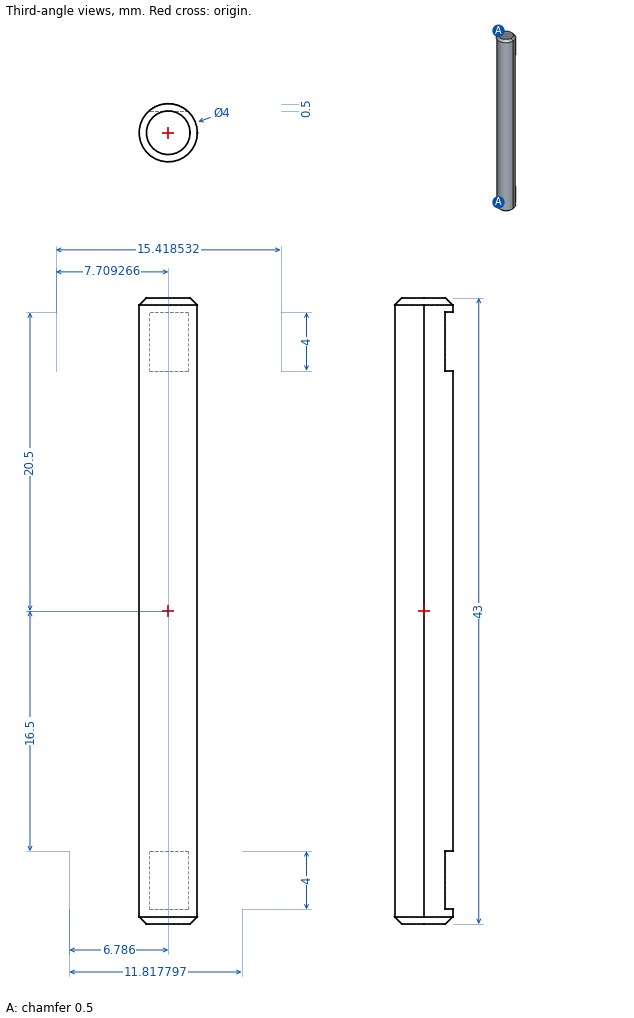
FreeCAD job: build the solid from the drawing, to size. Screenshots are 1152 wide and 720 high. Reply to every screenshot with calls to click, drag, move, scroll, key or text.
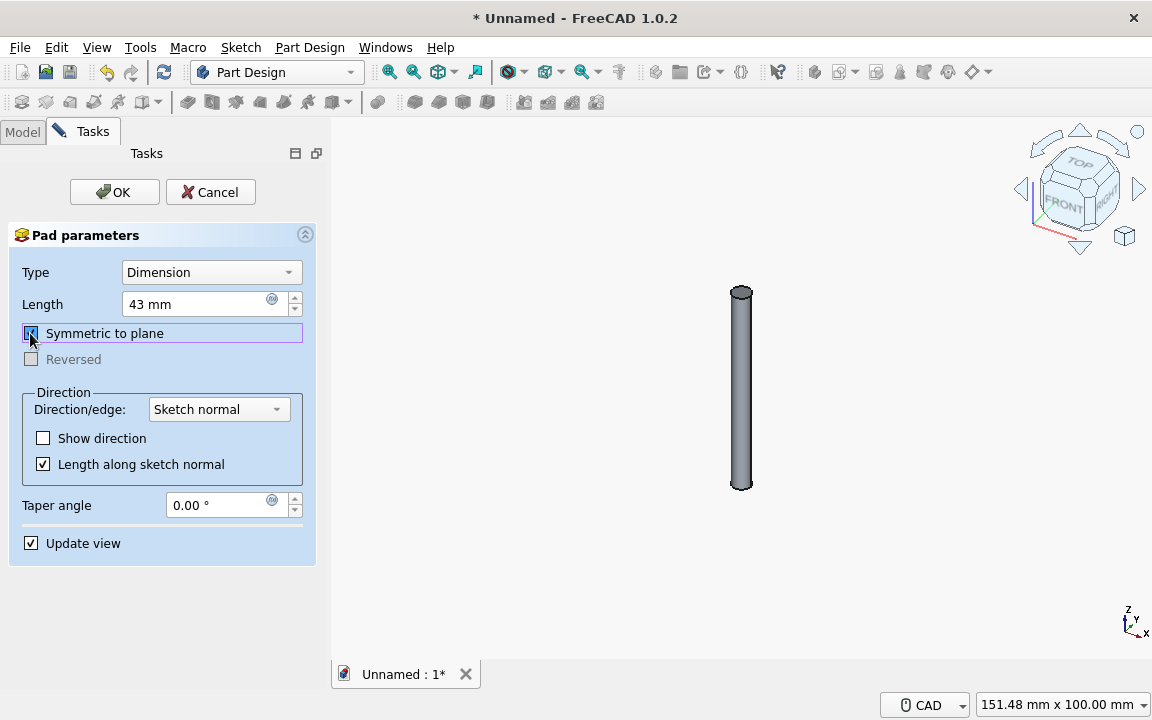
click(115, 192)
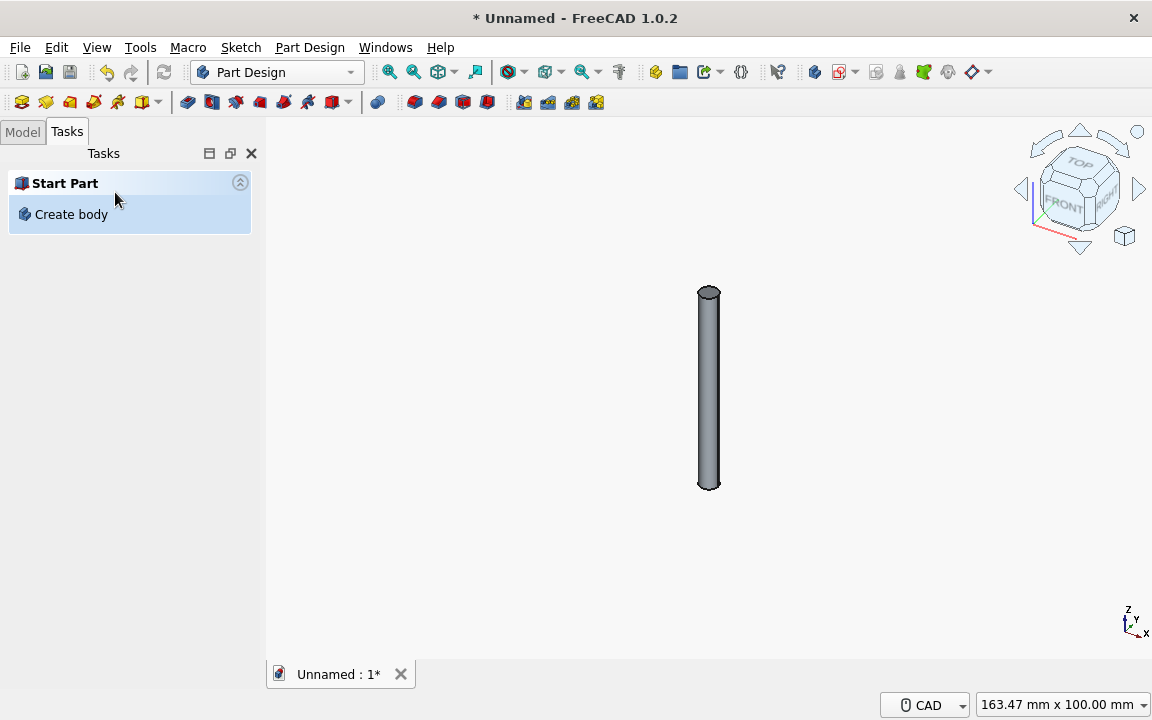
key(v)
key(f)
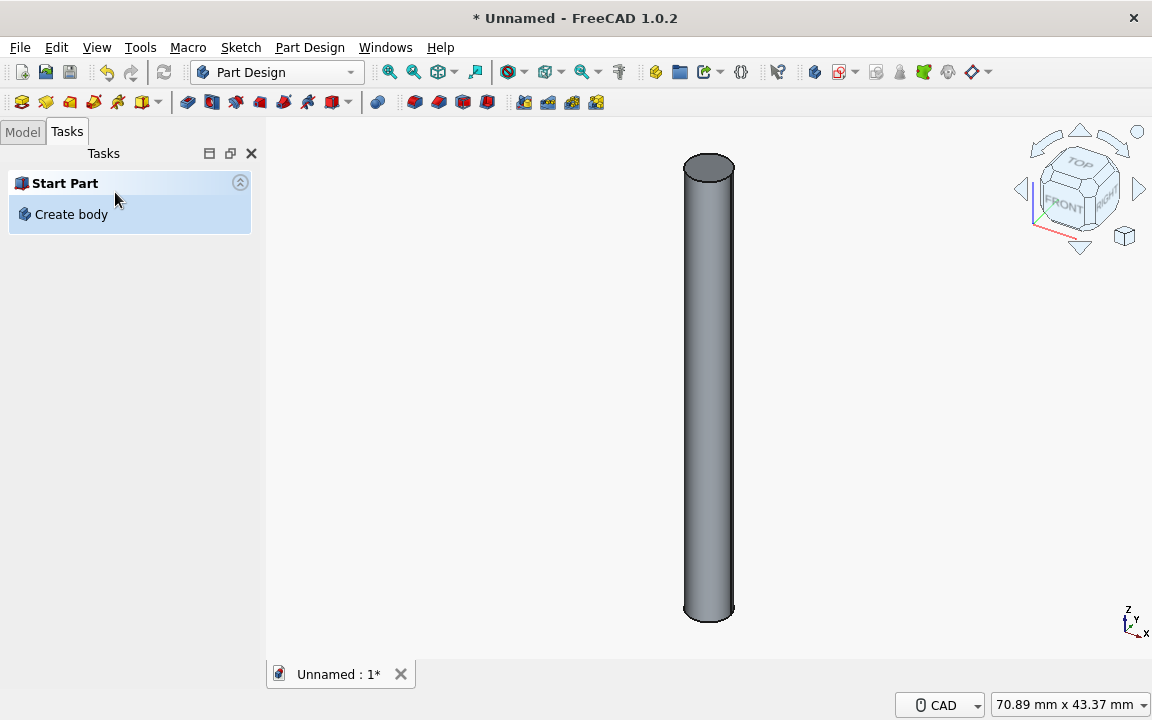
click(23, 131)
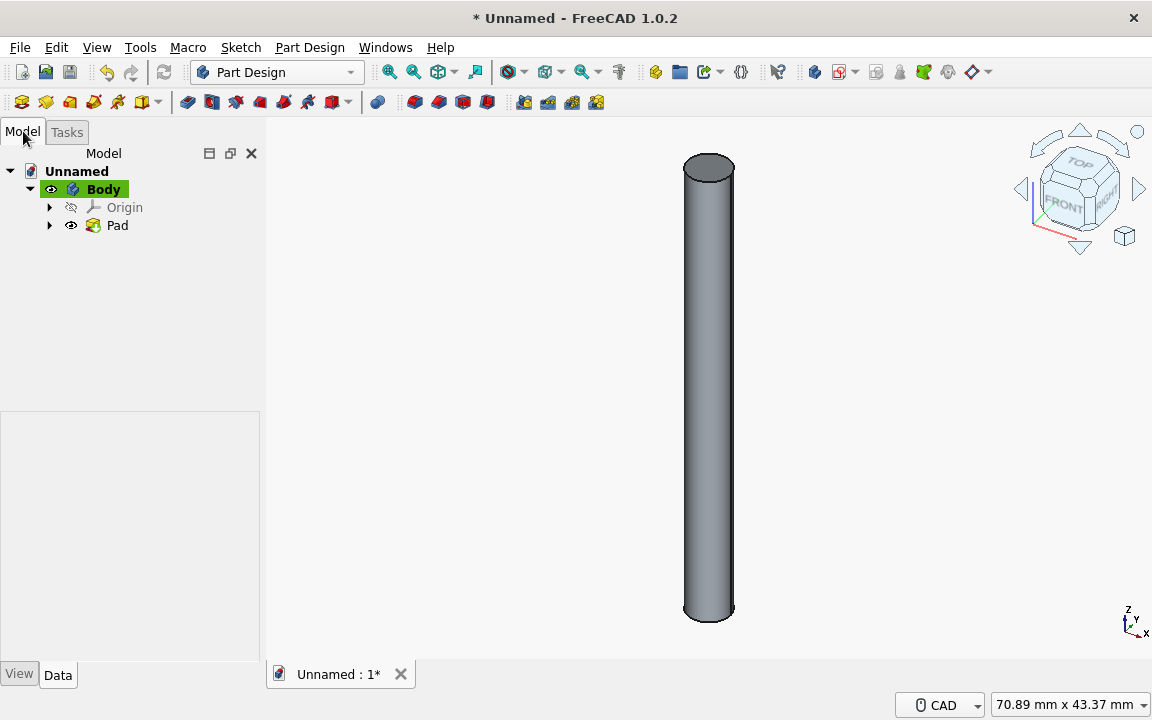
click(50, 207)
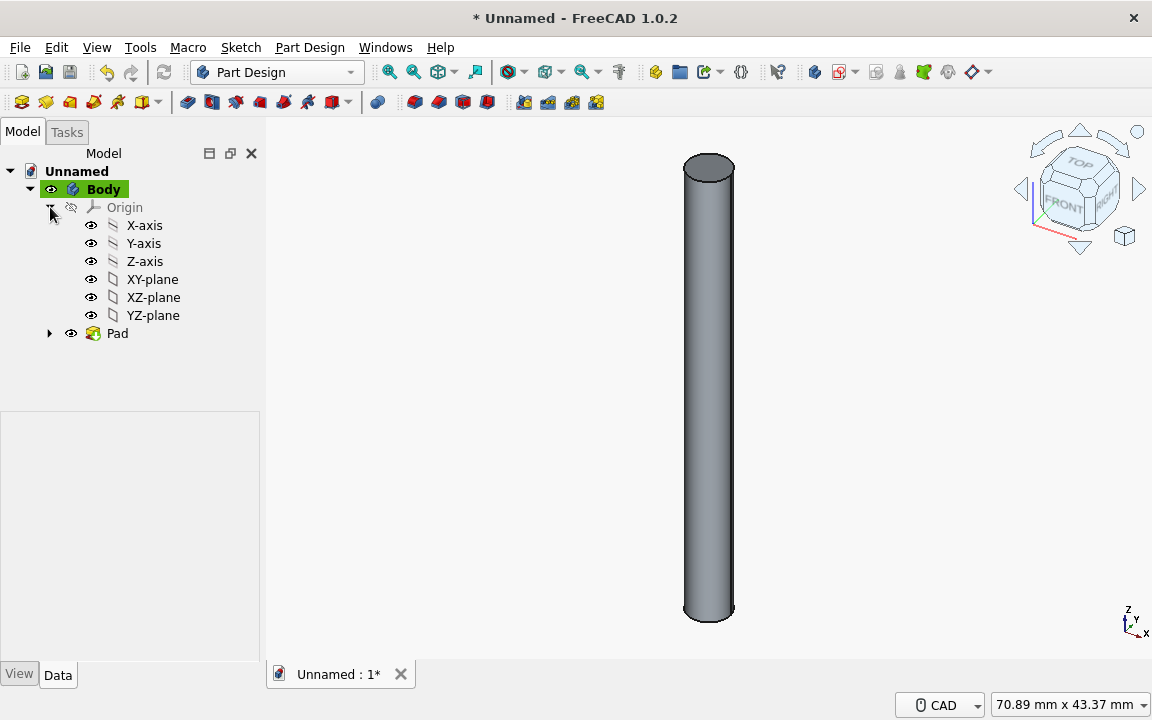
click(136, 297)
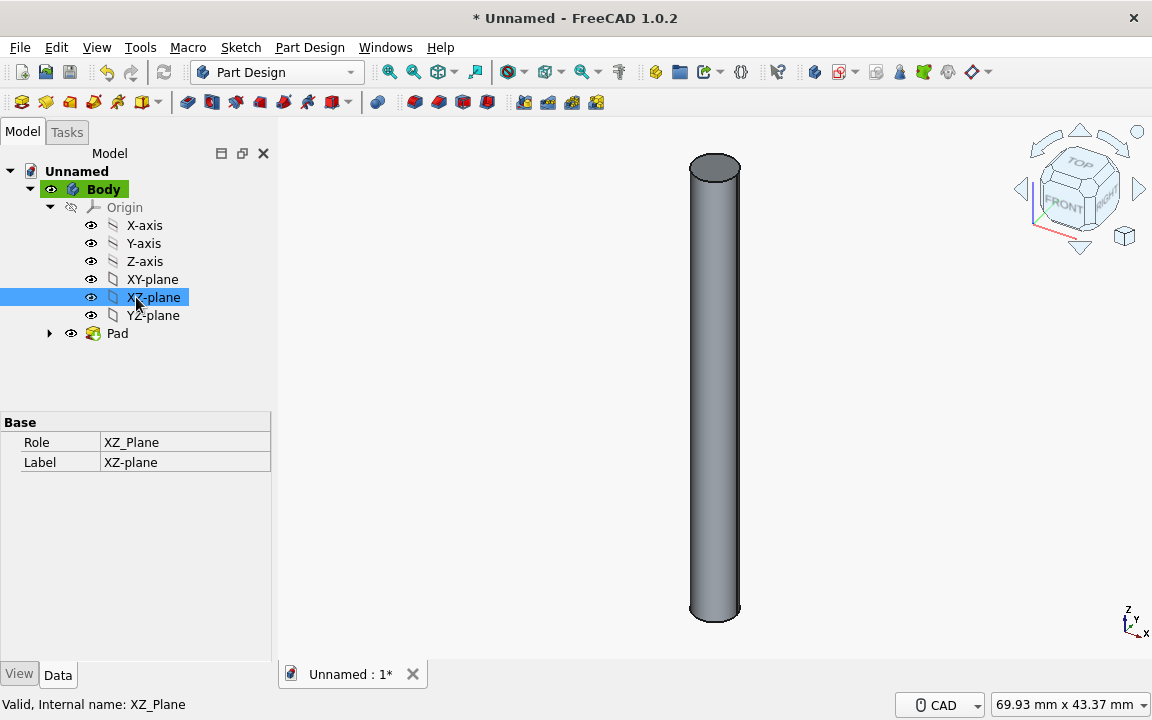
click(972, 72)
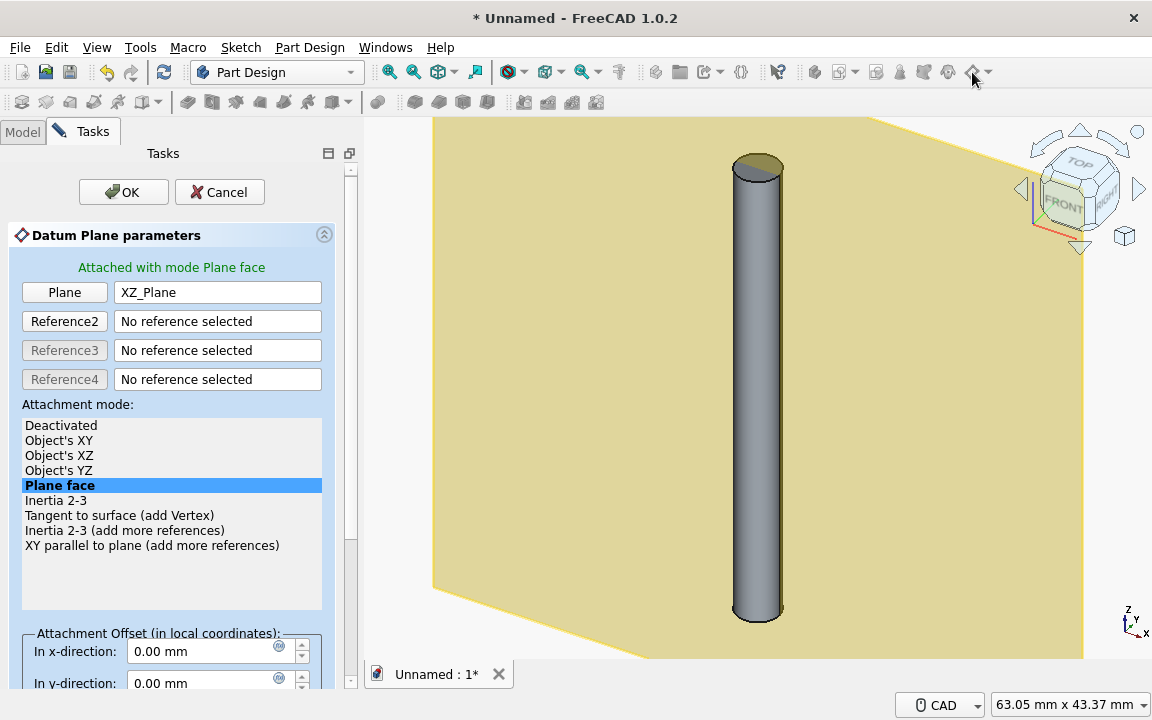
scroll(351, 426, down, 2)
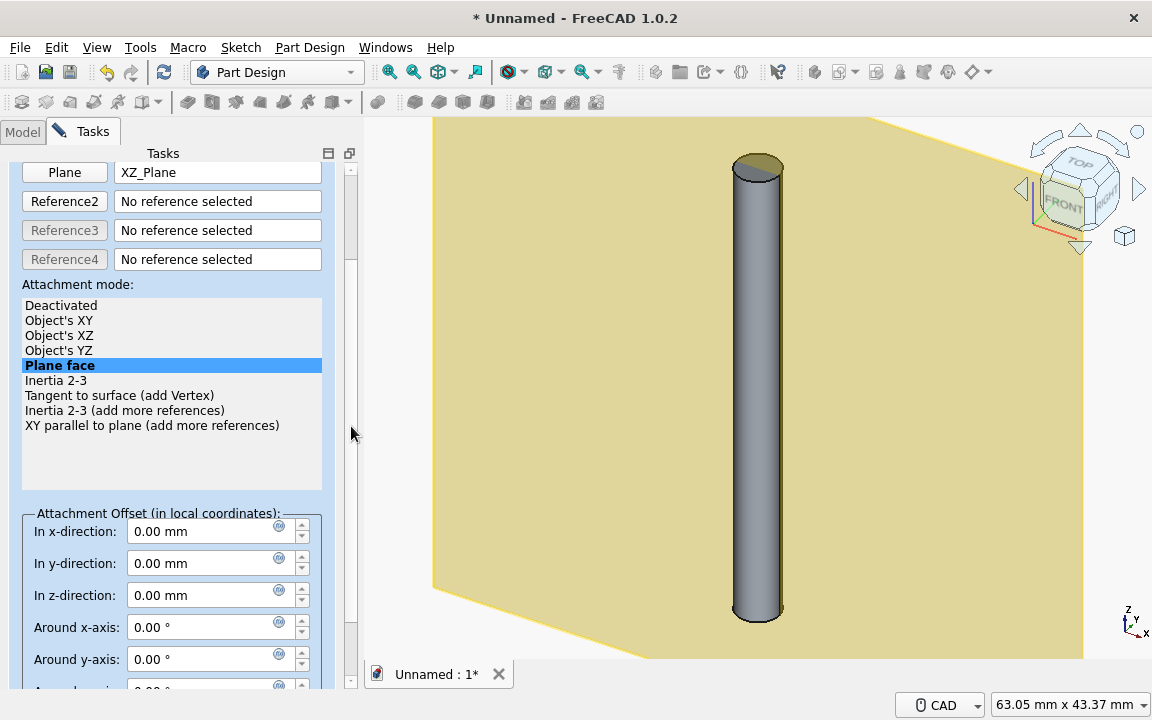
triple_click(210, 595)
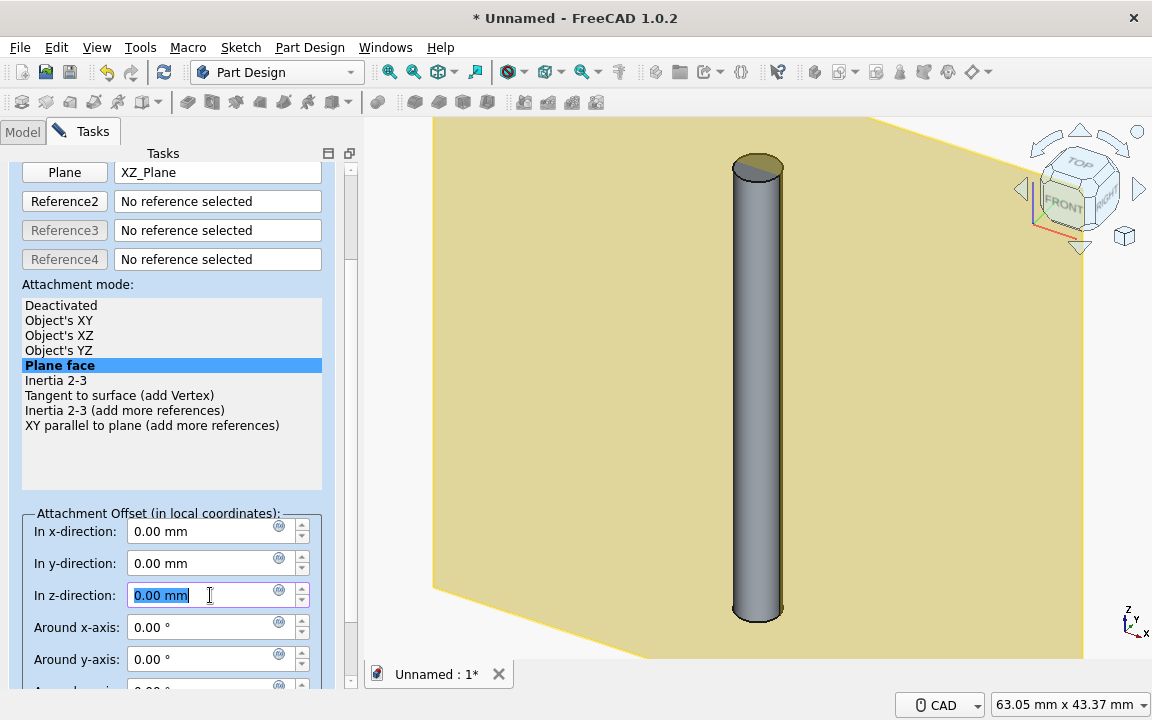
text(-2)
key(Tab)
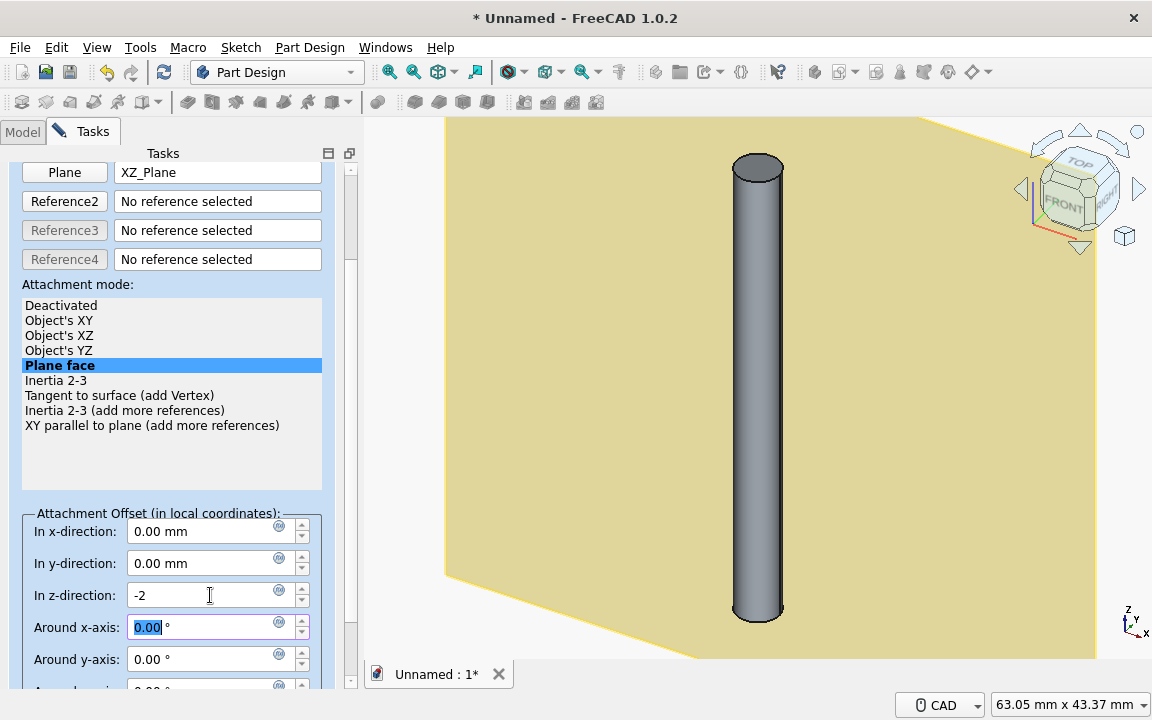
scroll(351, 426, up, 3)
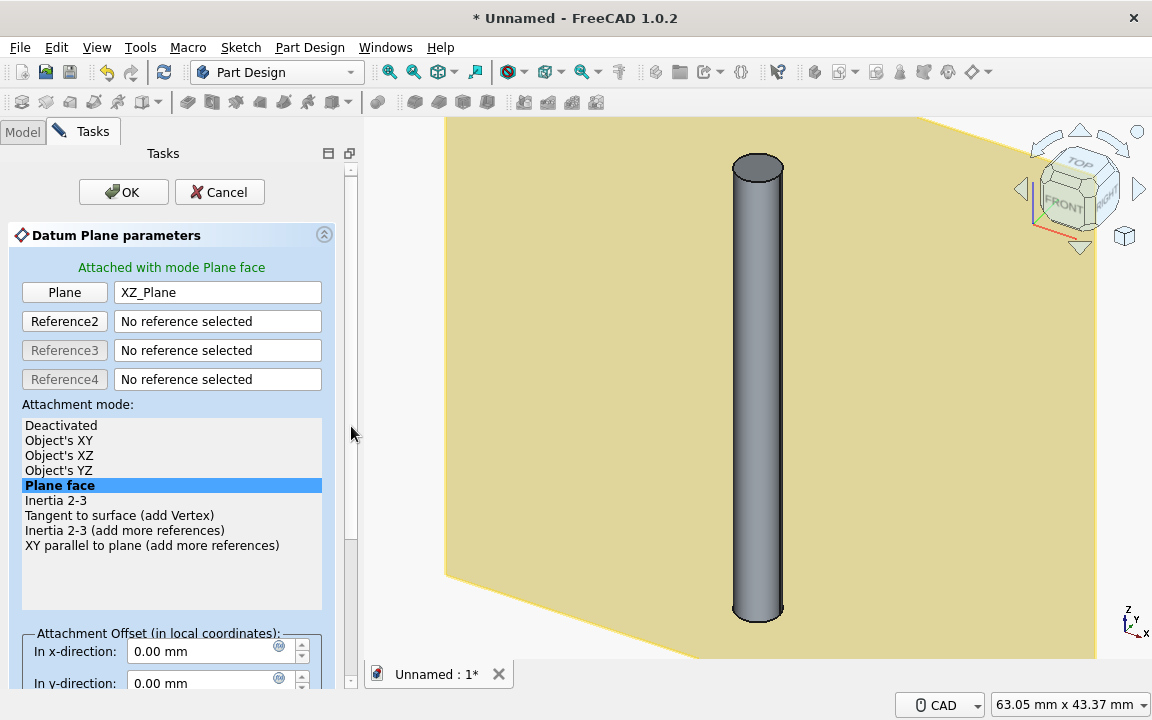
click(124, 192)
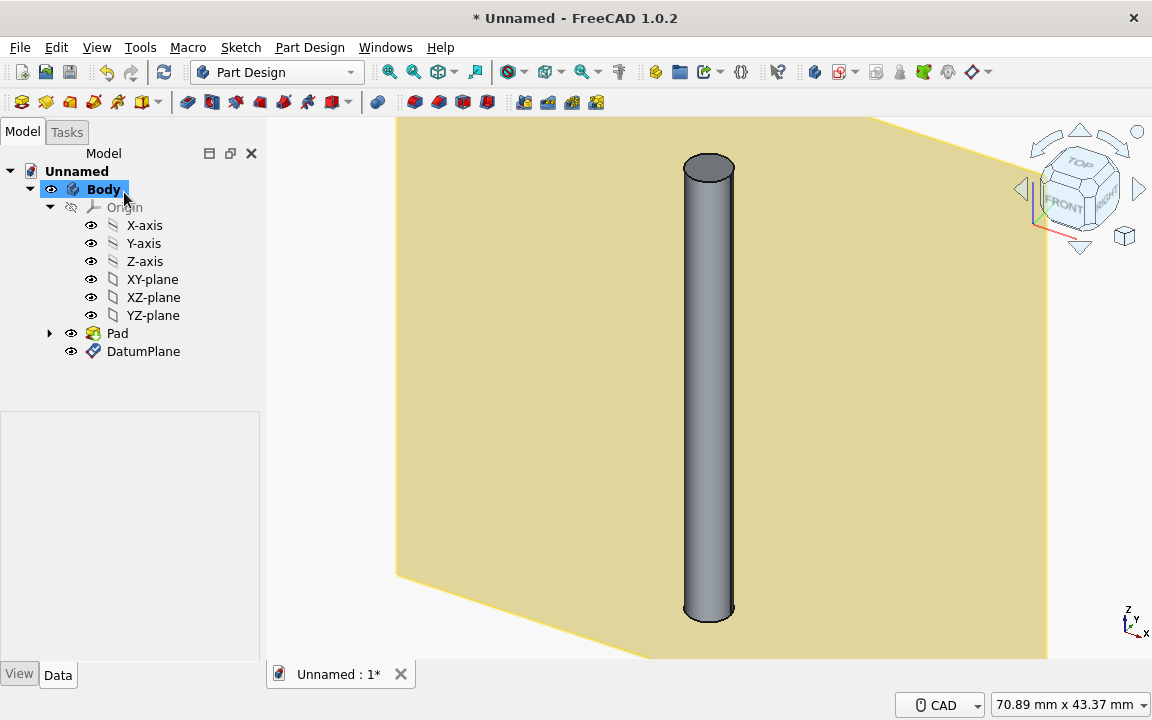
click(116, 351)